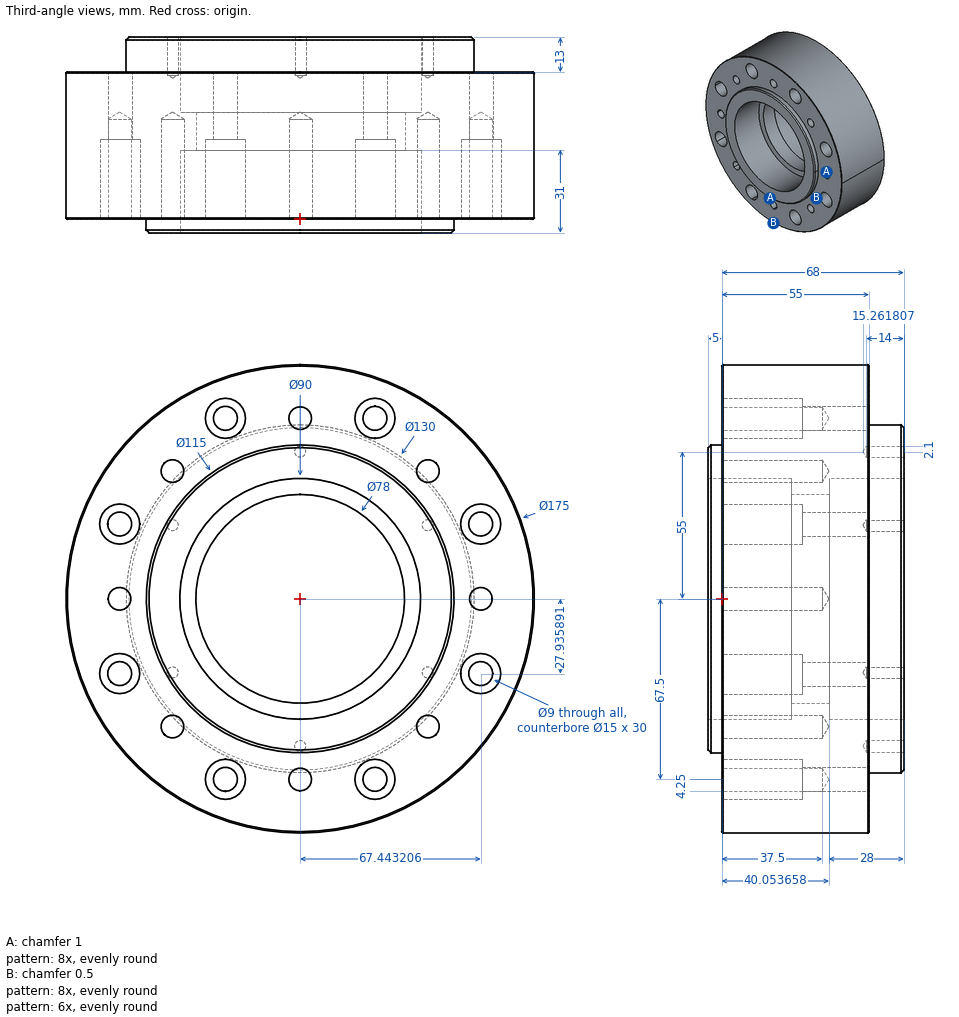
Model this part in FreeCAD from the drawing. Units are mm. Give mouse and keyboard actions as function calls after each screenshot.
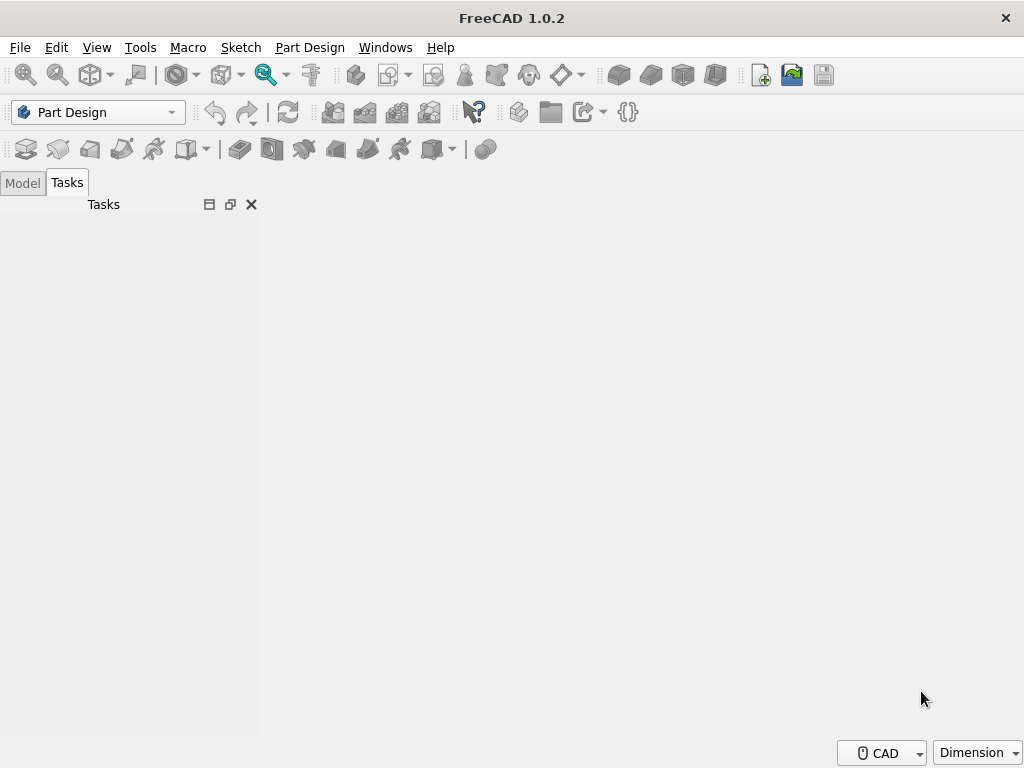
click(760, 76)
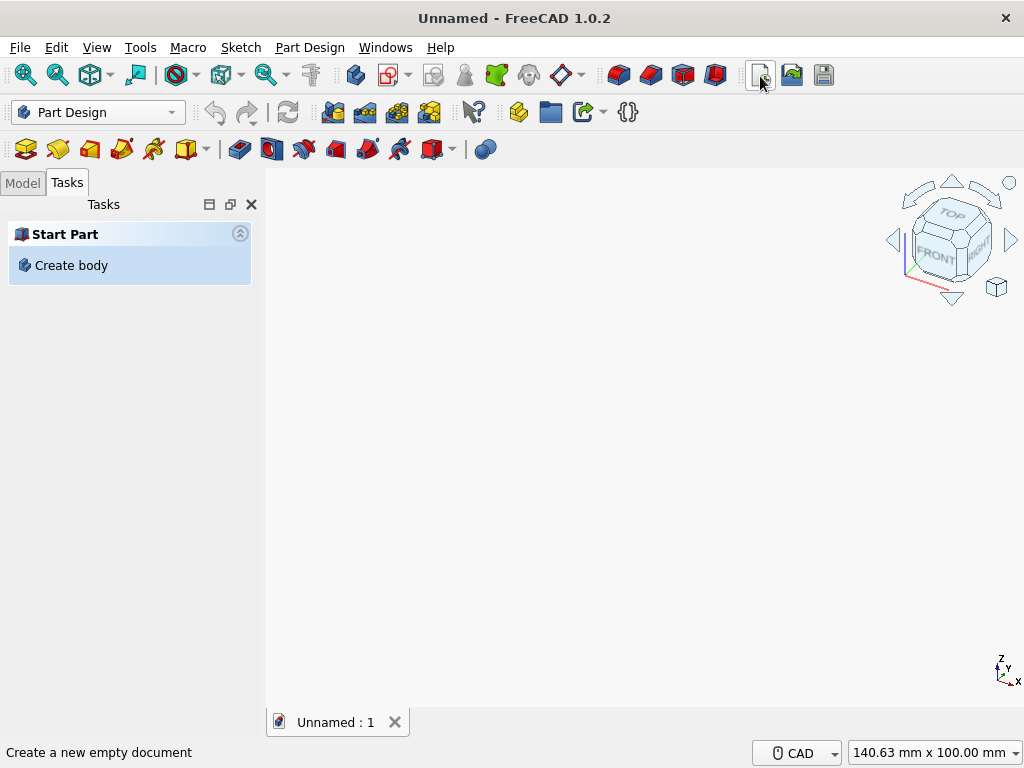
click(388, 76)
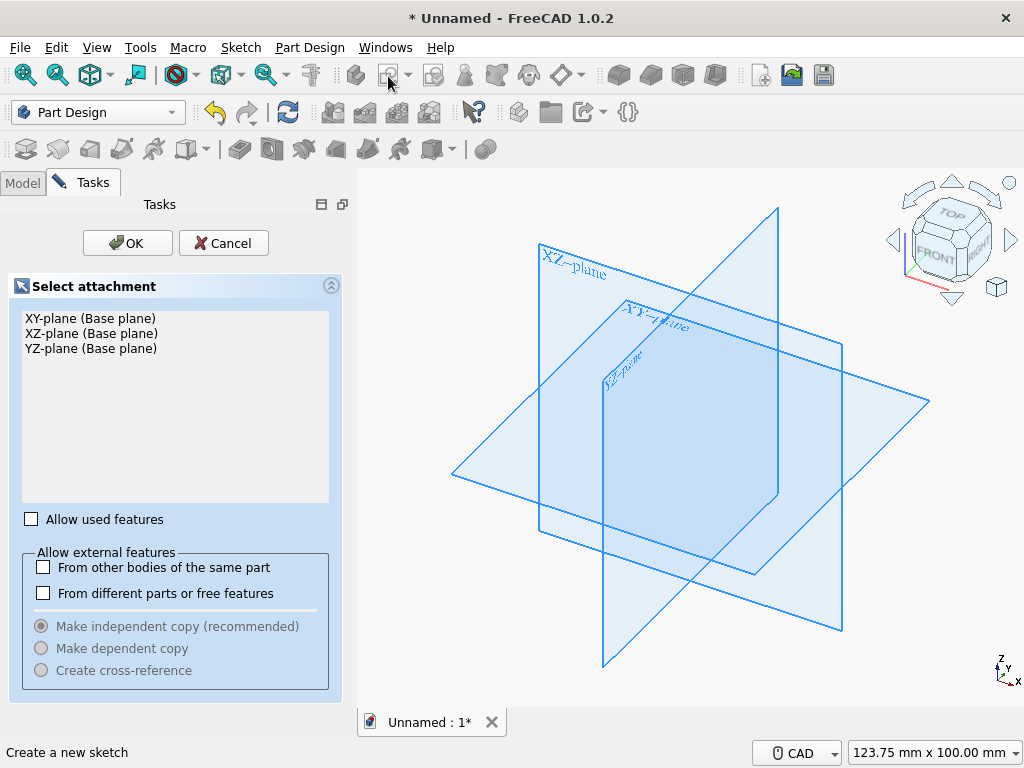
click(82, 334)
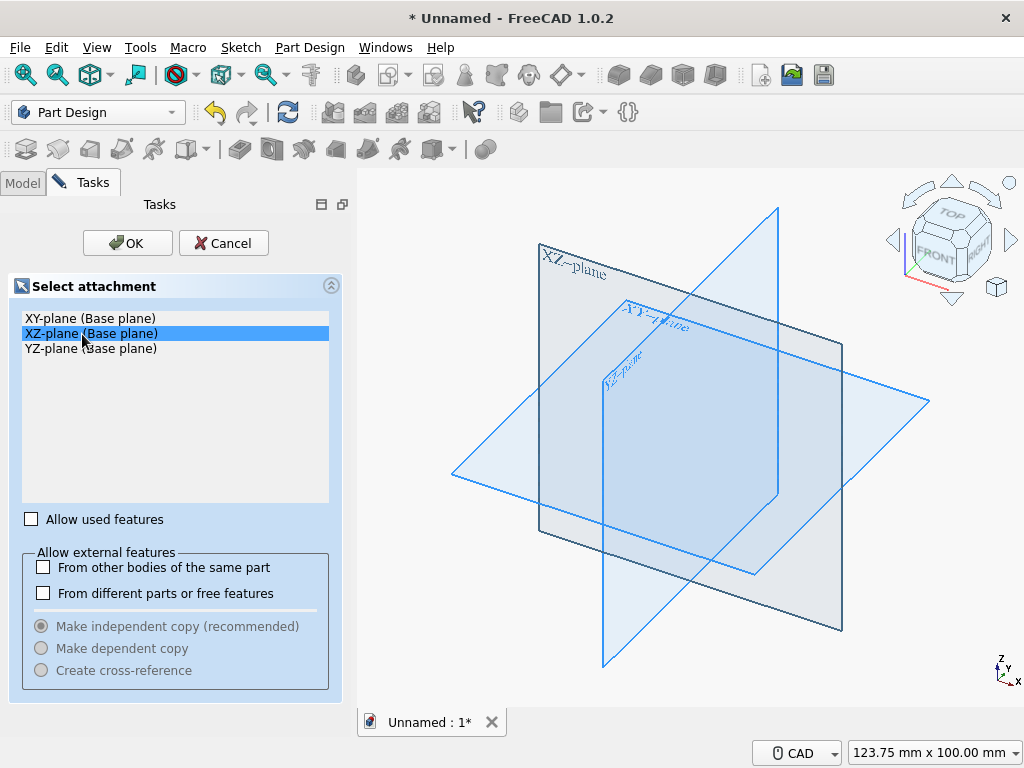
click(128, 243)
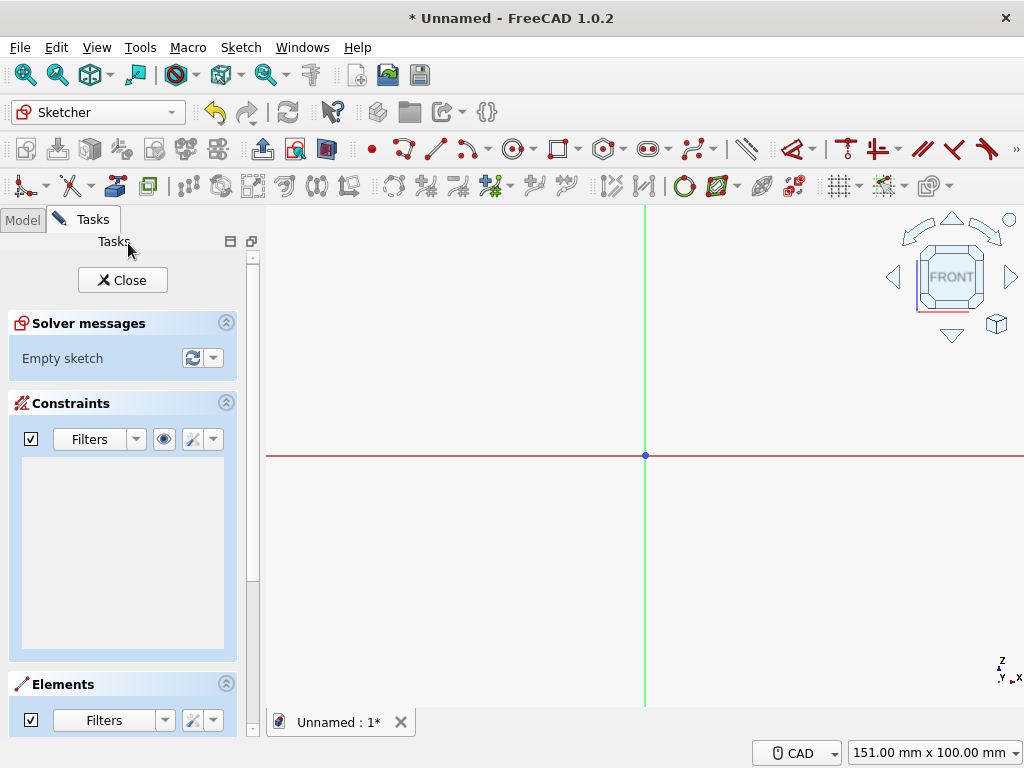
scroll(537, 456, down, 5)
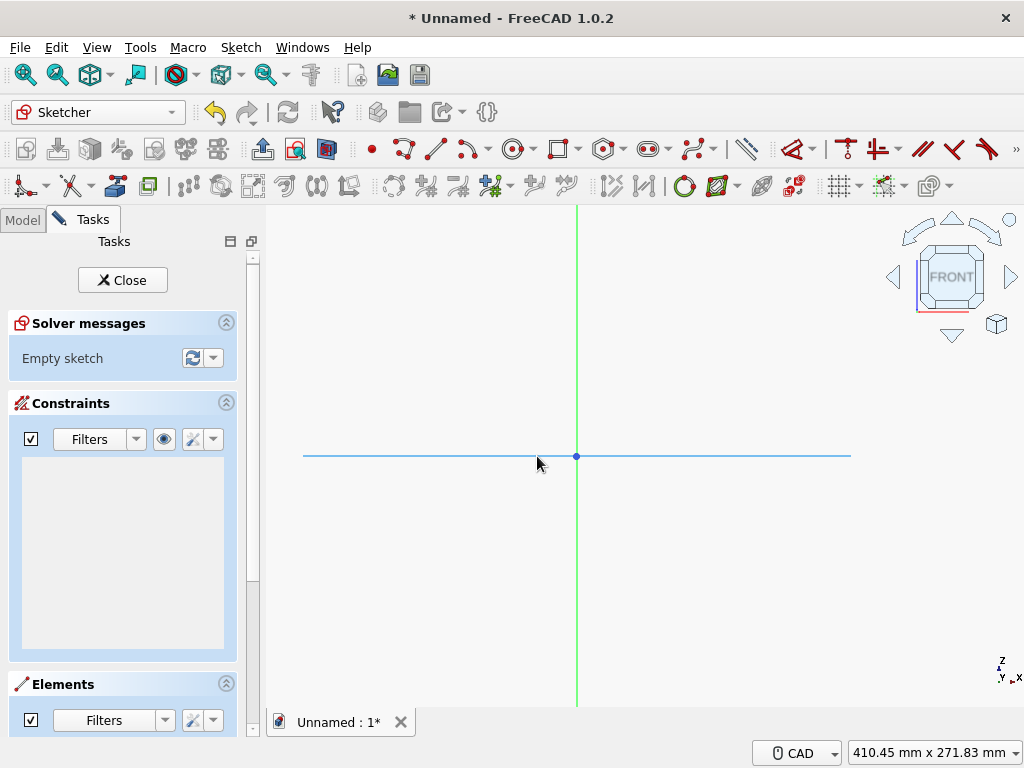
click(514, 150)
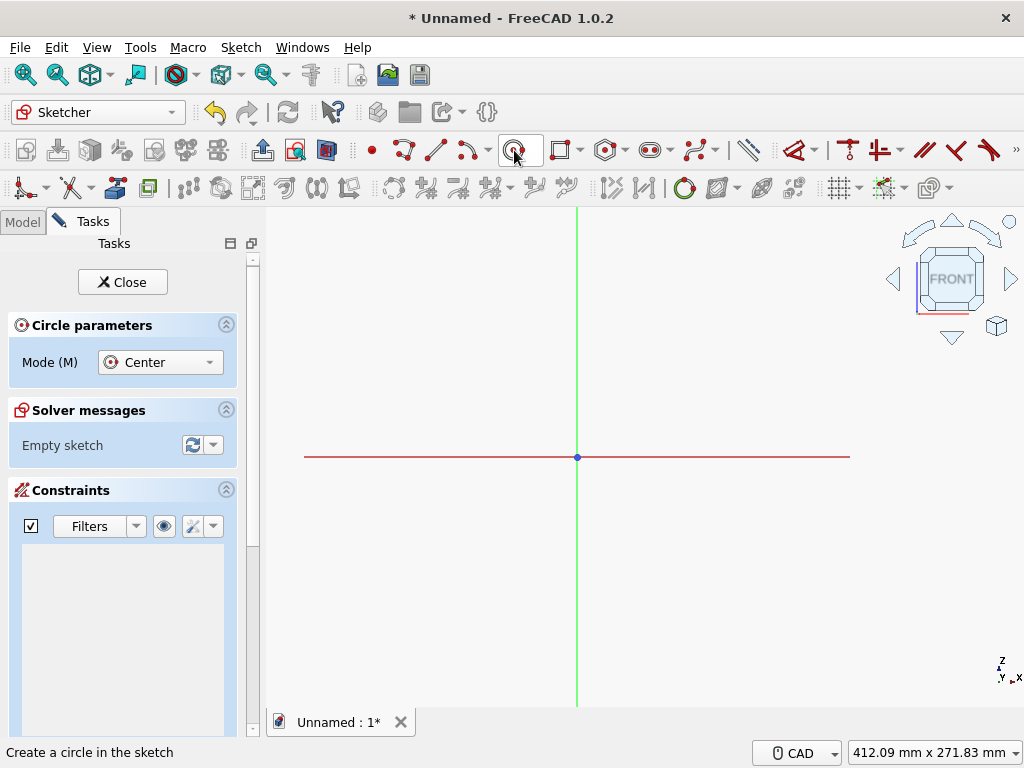
click(577, 457)
click(691, 344)
key(Escape)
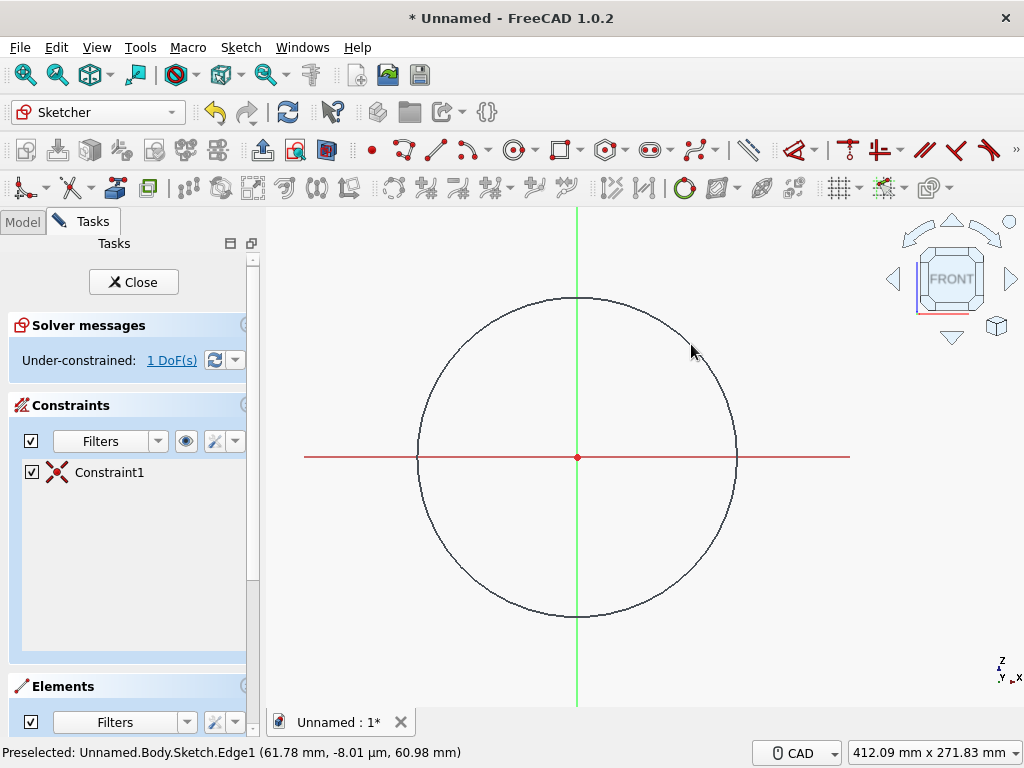
click(794, 150)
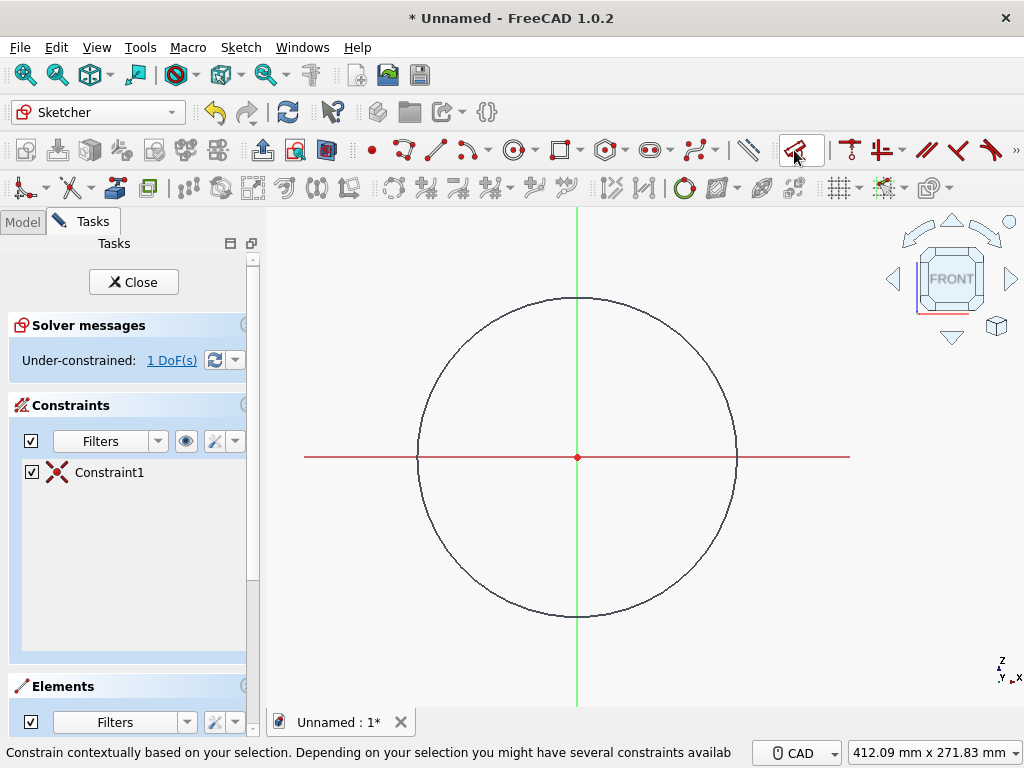
click(690, 344)
click(713, 321)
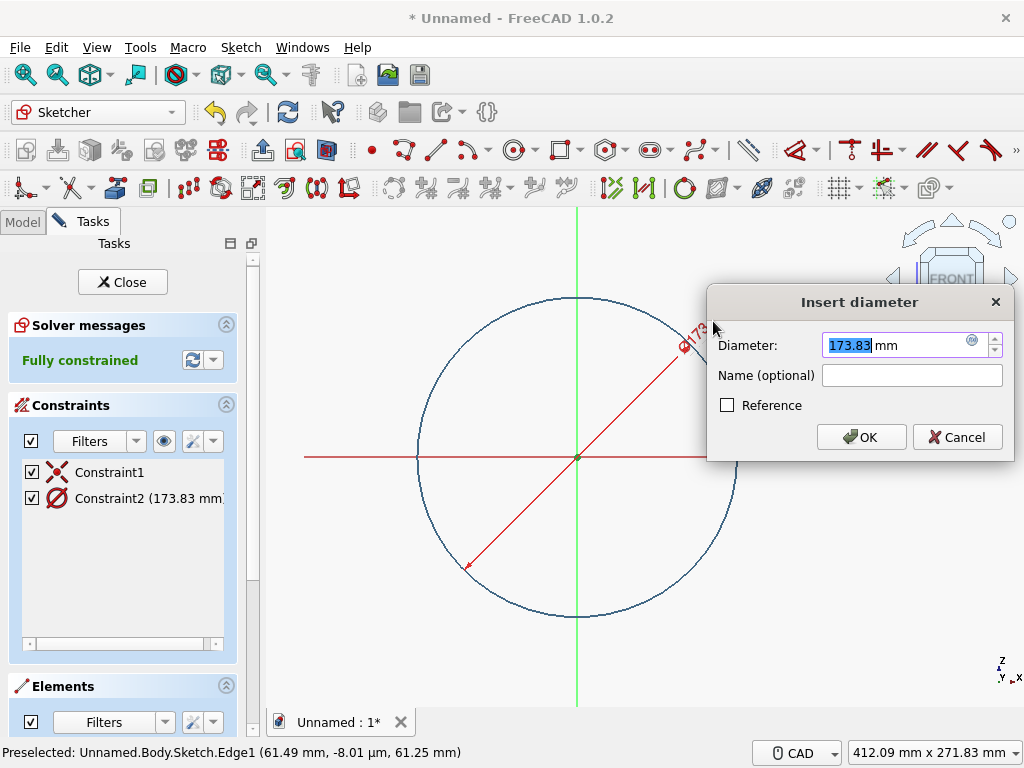
text(175)
key(Return)
key(Escape)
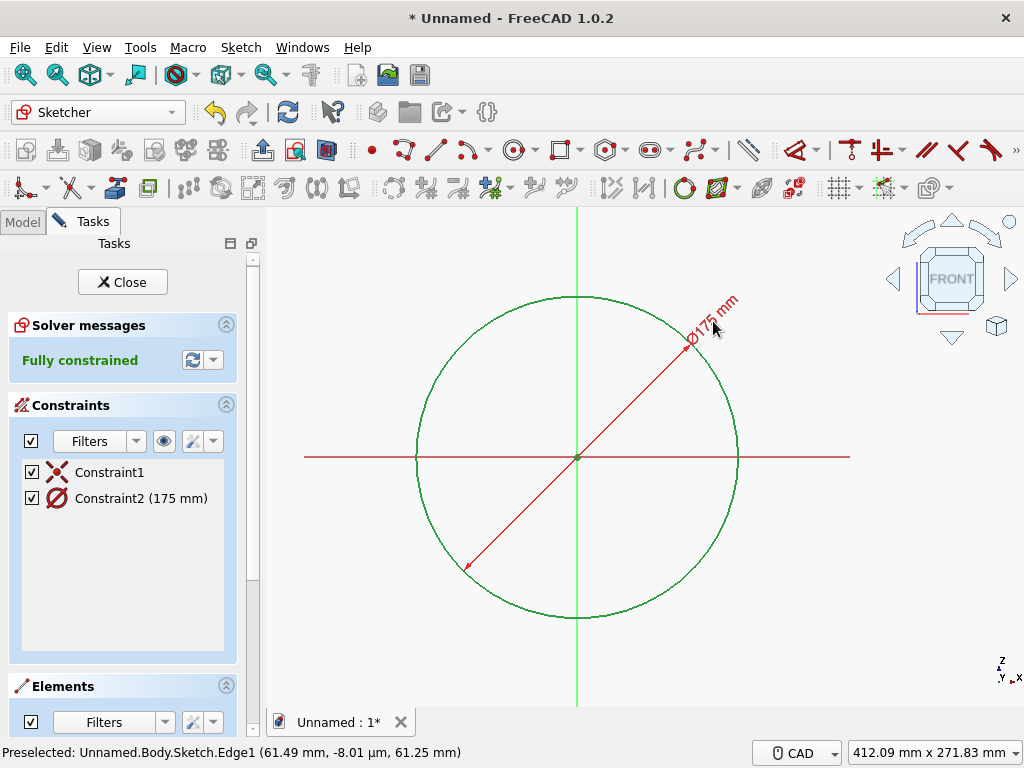
click(123, 282)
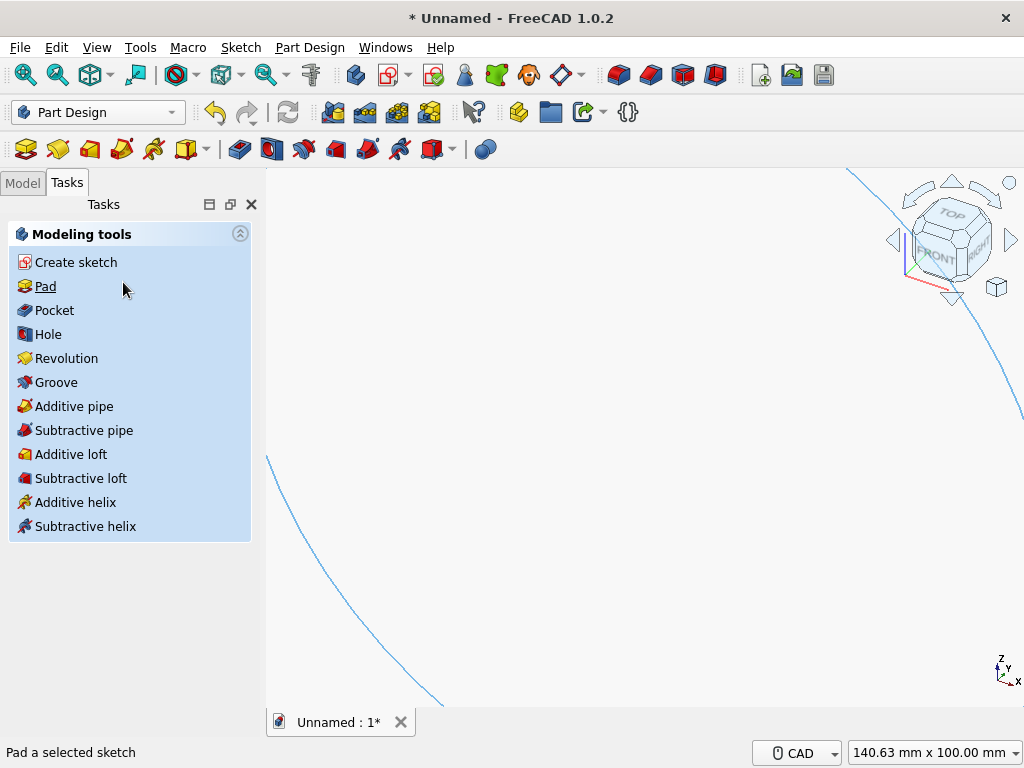
click(26, 150)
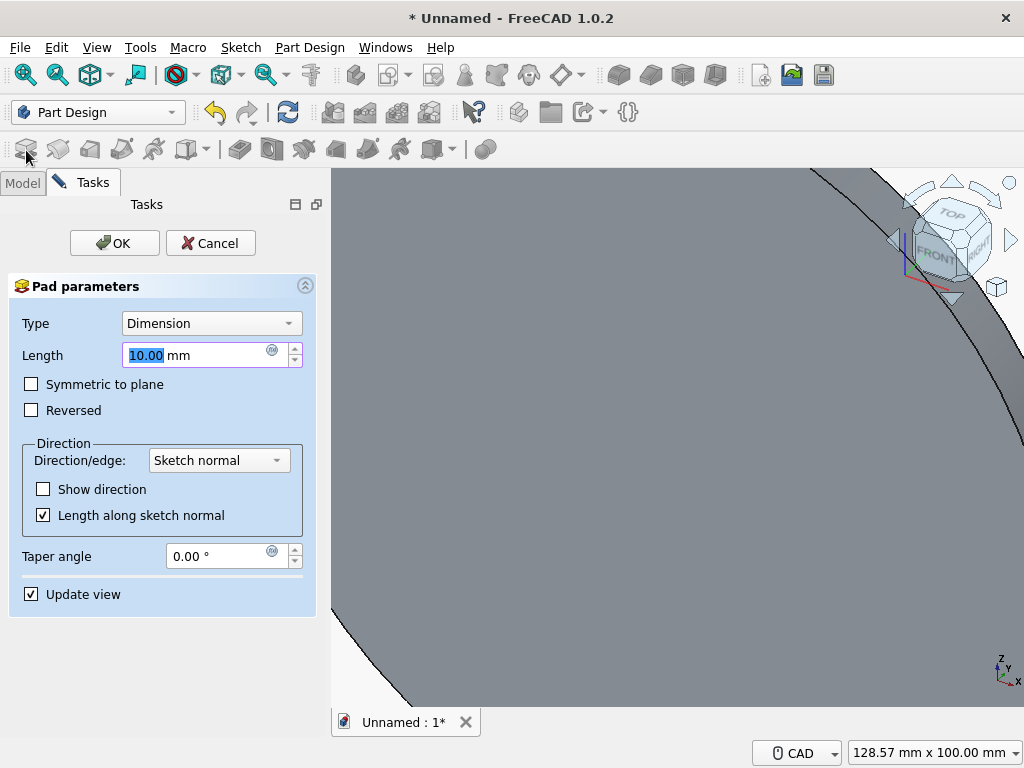
text(55)
key(Tab)